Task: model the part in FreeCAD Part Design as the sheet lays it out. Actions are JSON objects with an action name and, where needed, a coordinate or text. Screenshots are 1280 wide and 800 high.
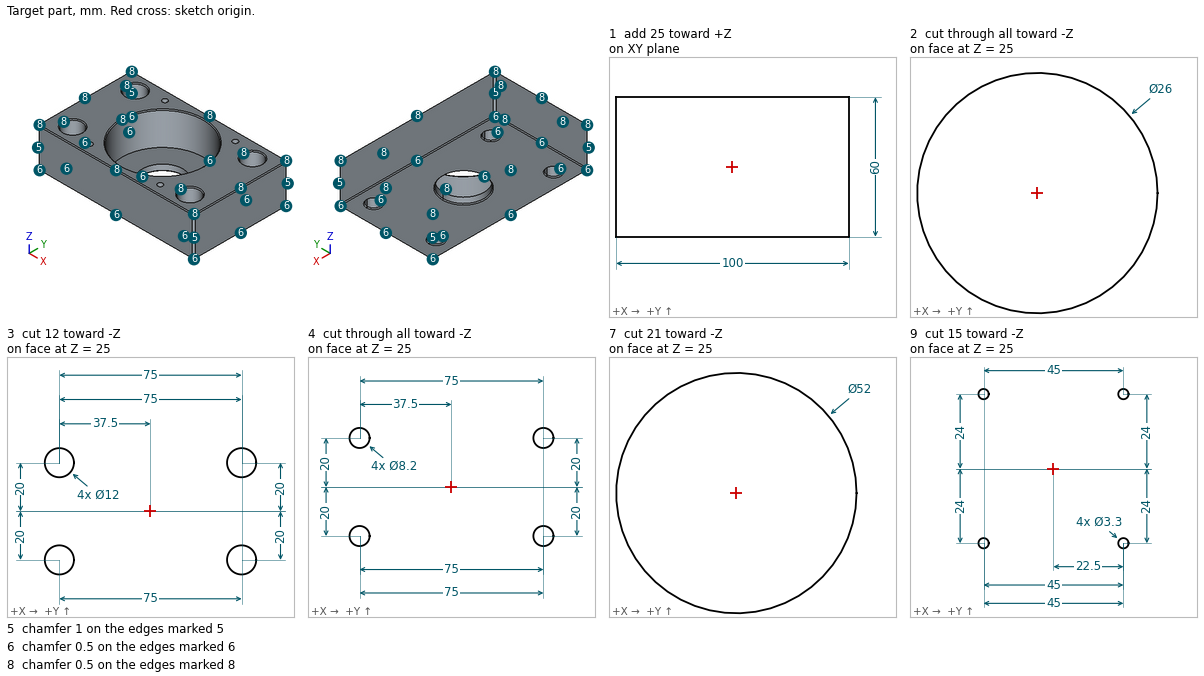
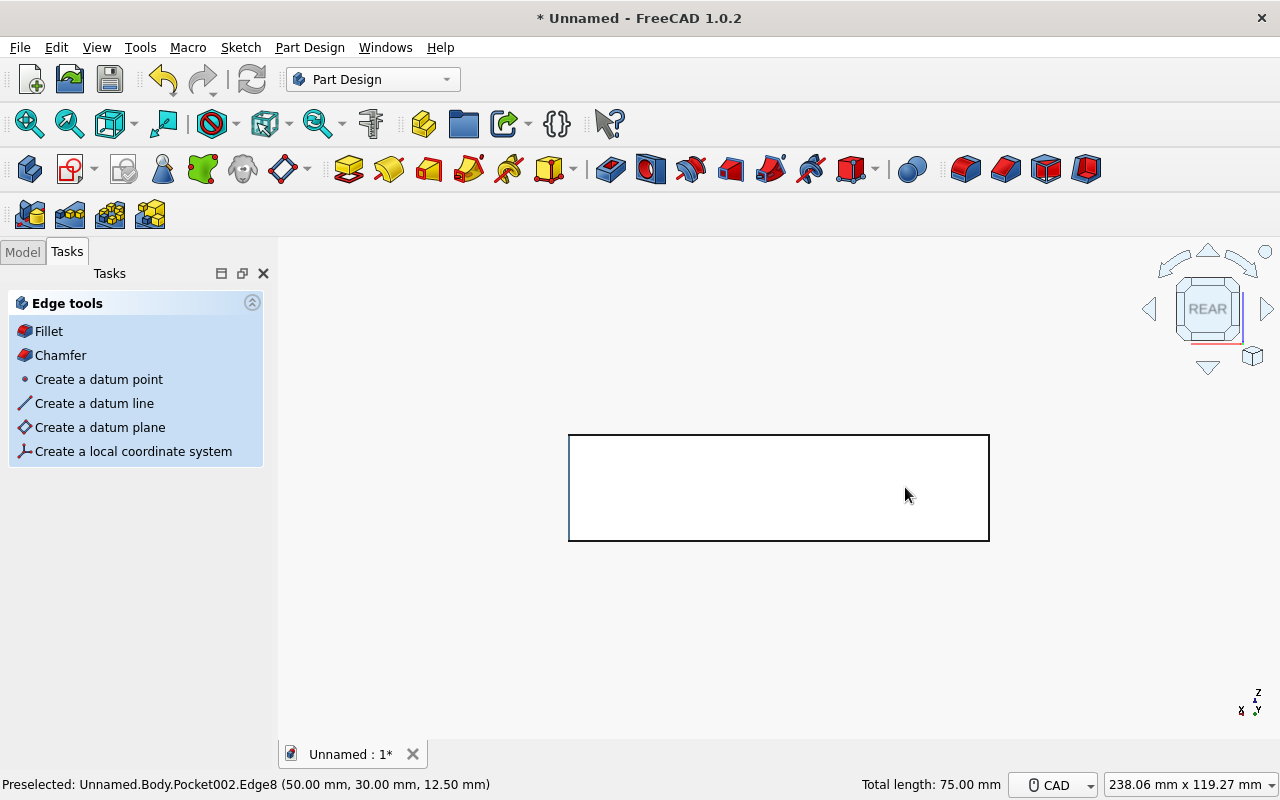
{"action": "key", "text": "v f"}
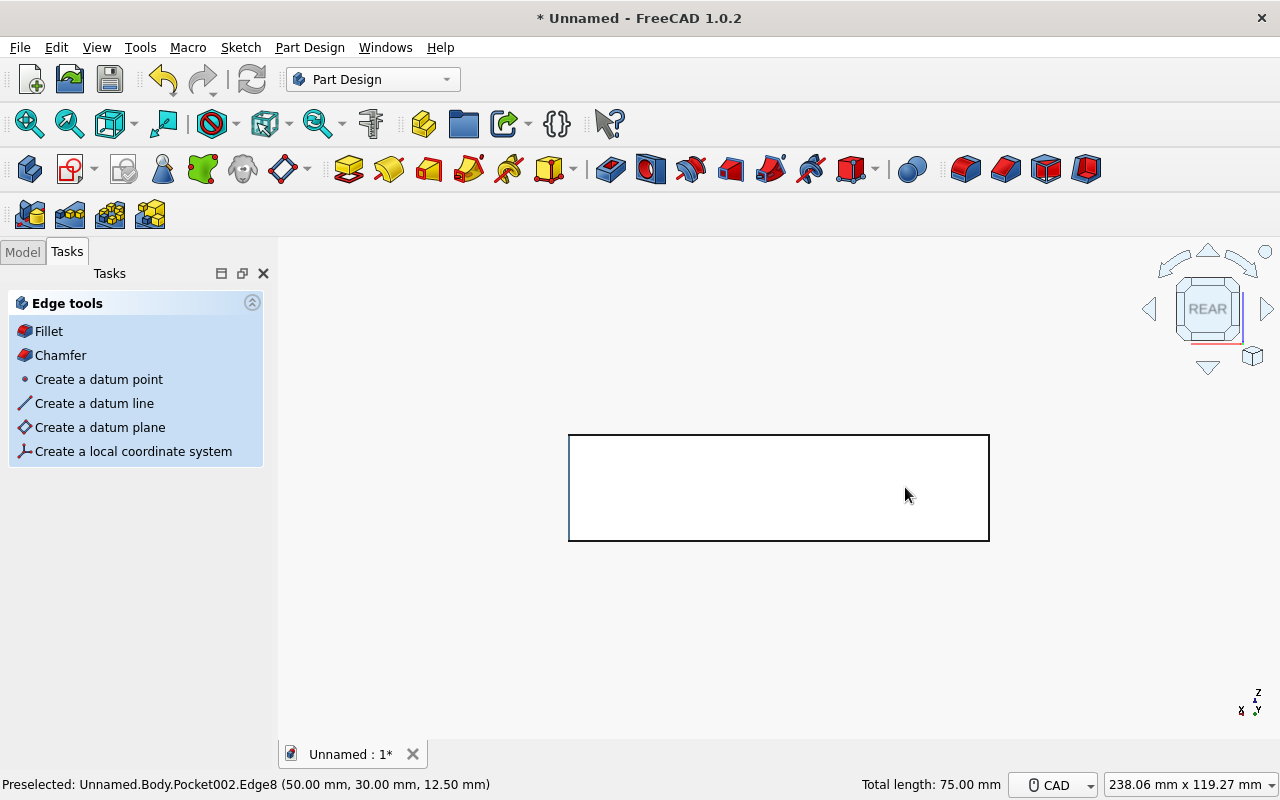
{"action": "left_click", "coordinate": [989, 487], "text": "ctrl"}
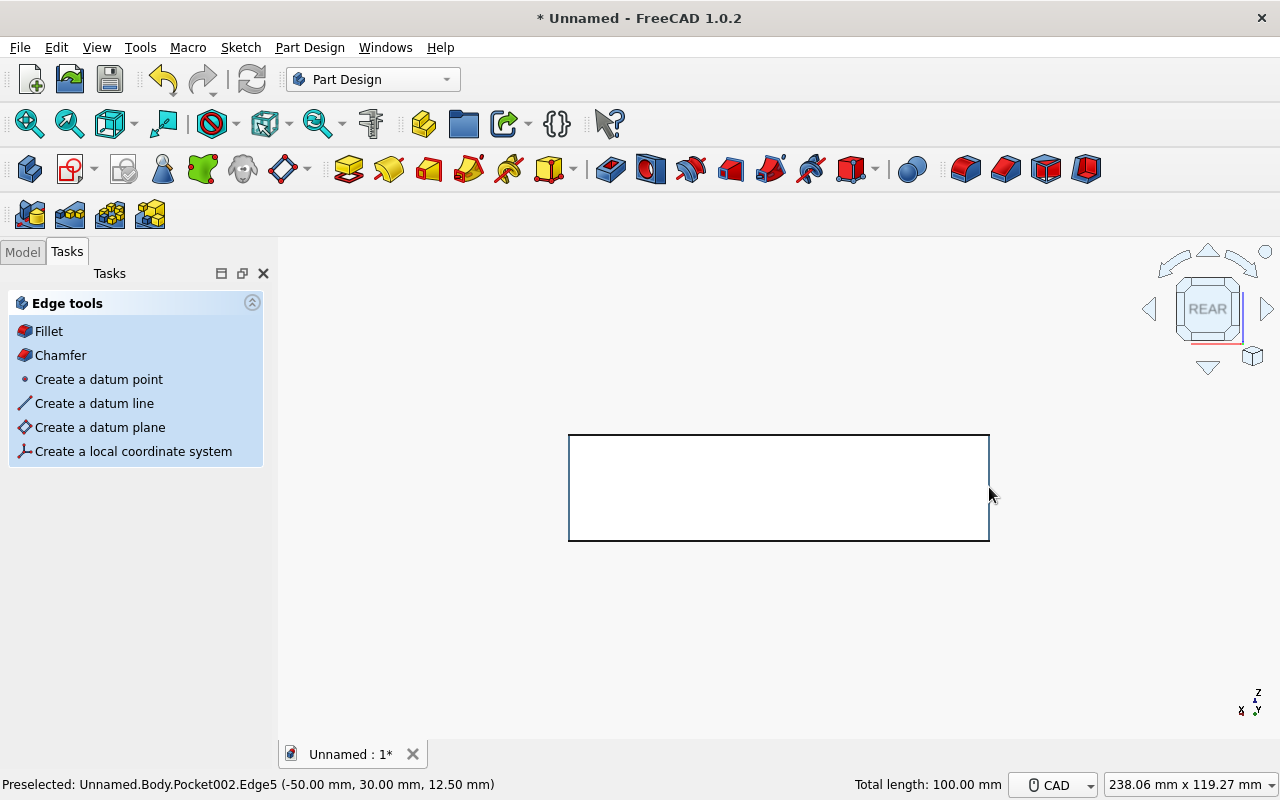
{"action": "left_click", "coordinate": [1006, 170]}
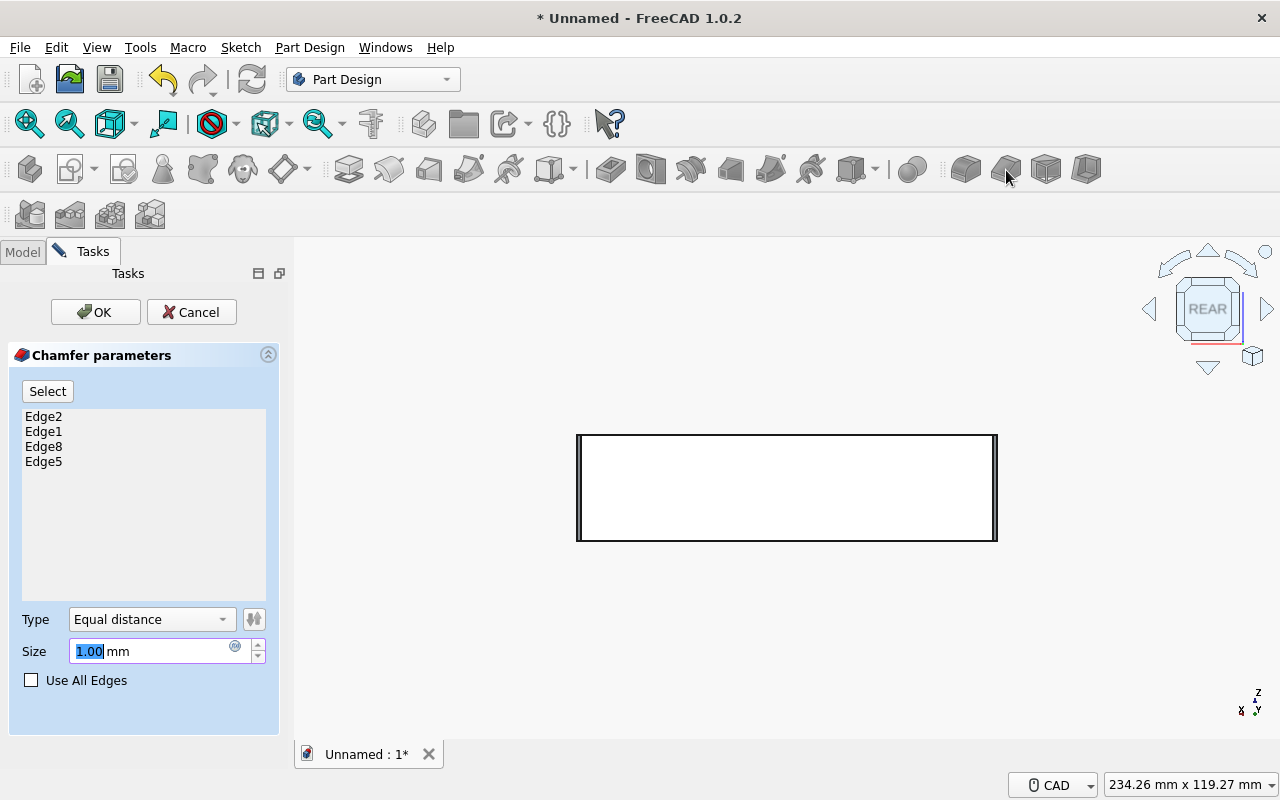
{"action": "type", "text": "1"}
{"action": "key", "text": "Tab"}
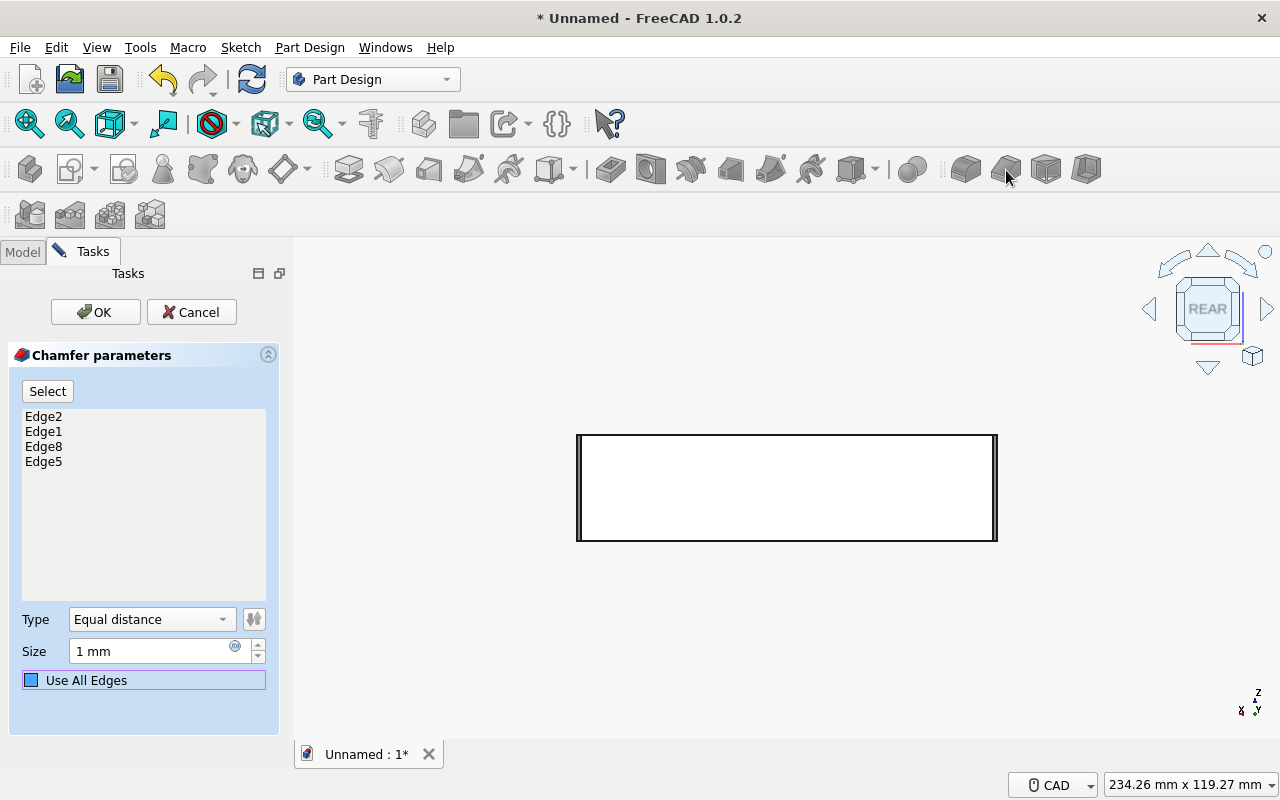
{"action": "left_click", "coordinate": [96, 312]}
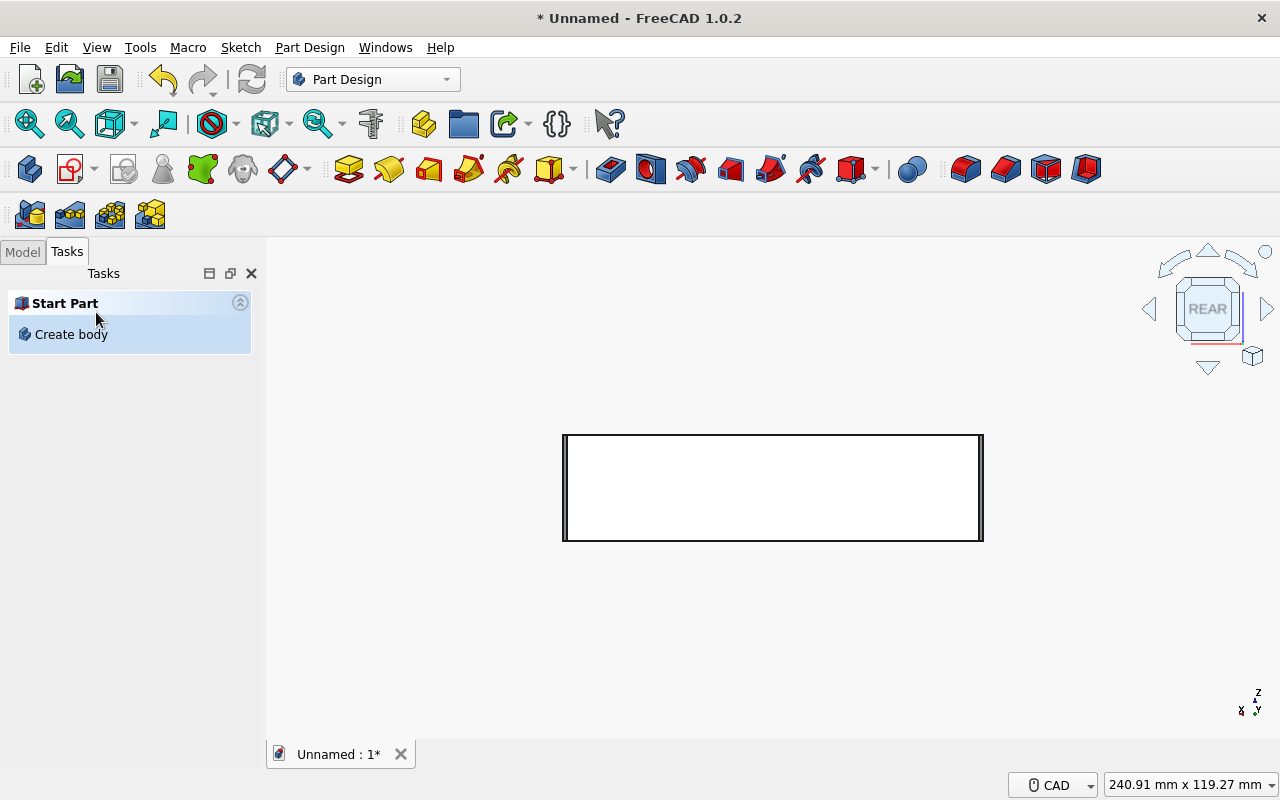
{"action": "left_click", "coordinate": [30, 124]}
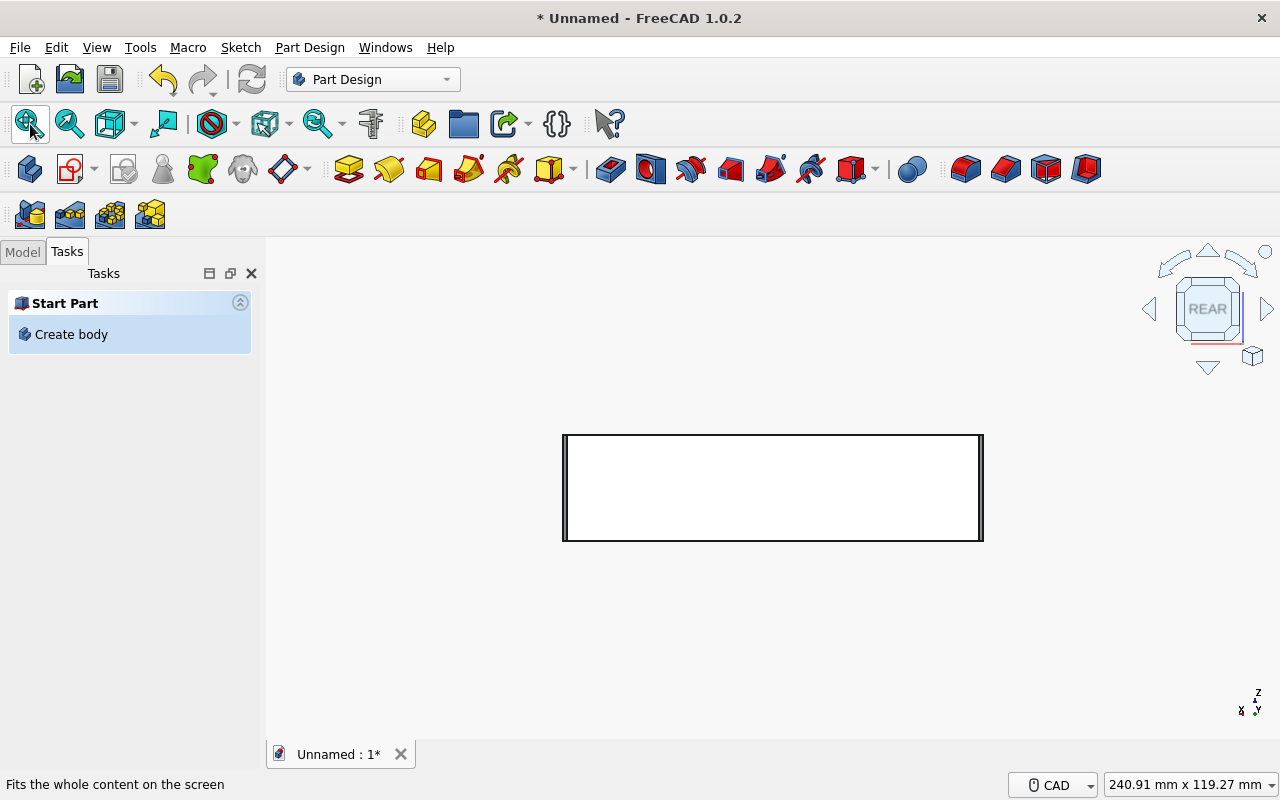
{"action": "key", "text": "0"}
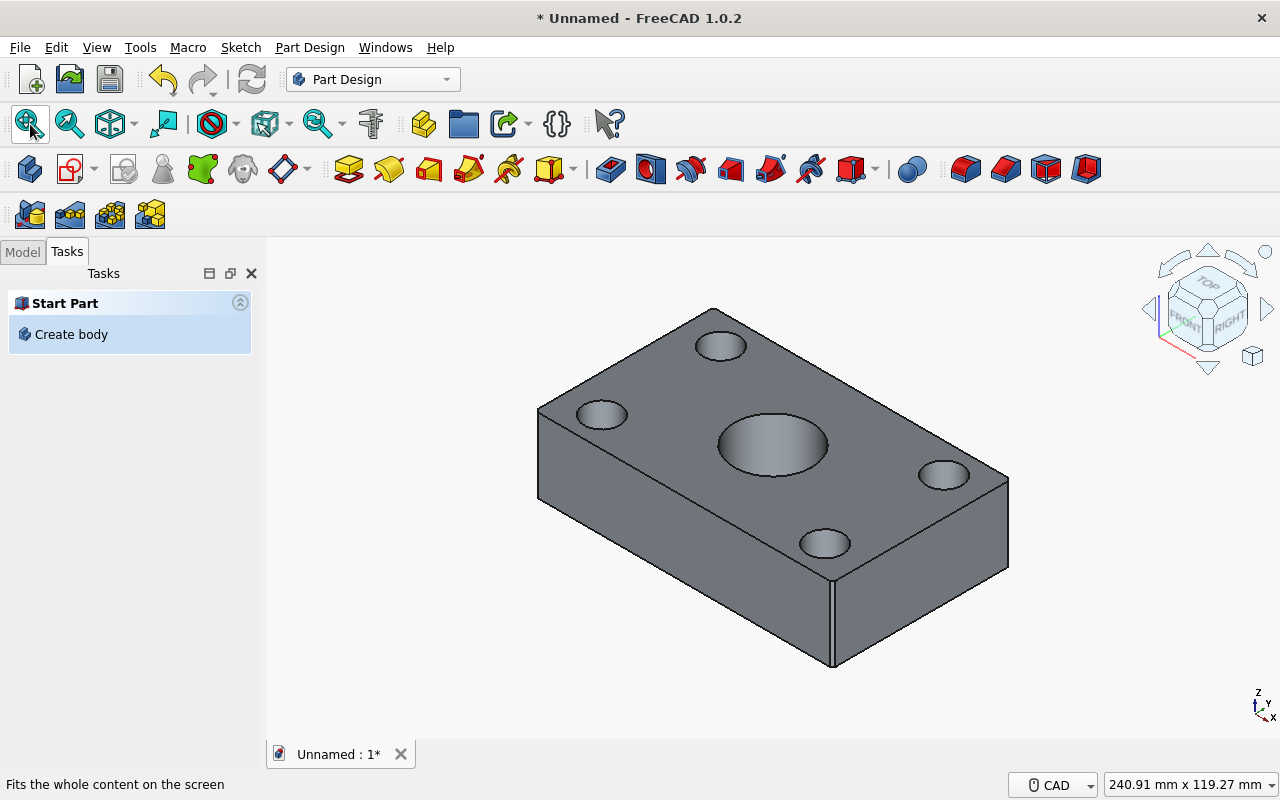
{"action": "key", "text": "2"}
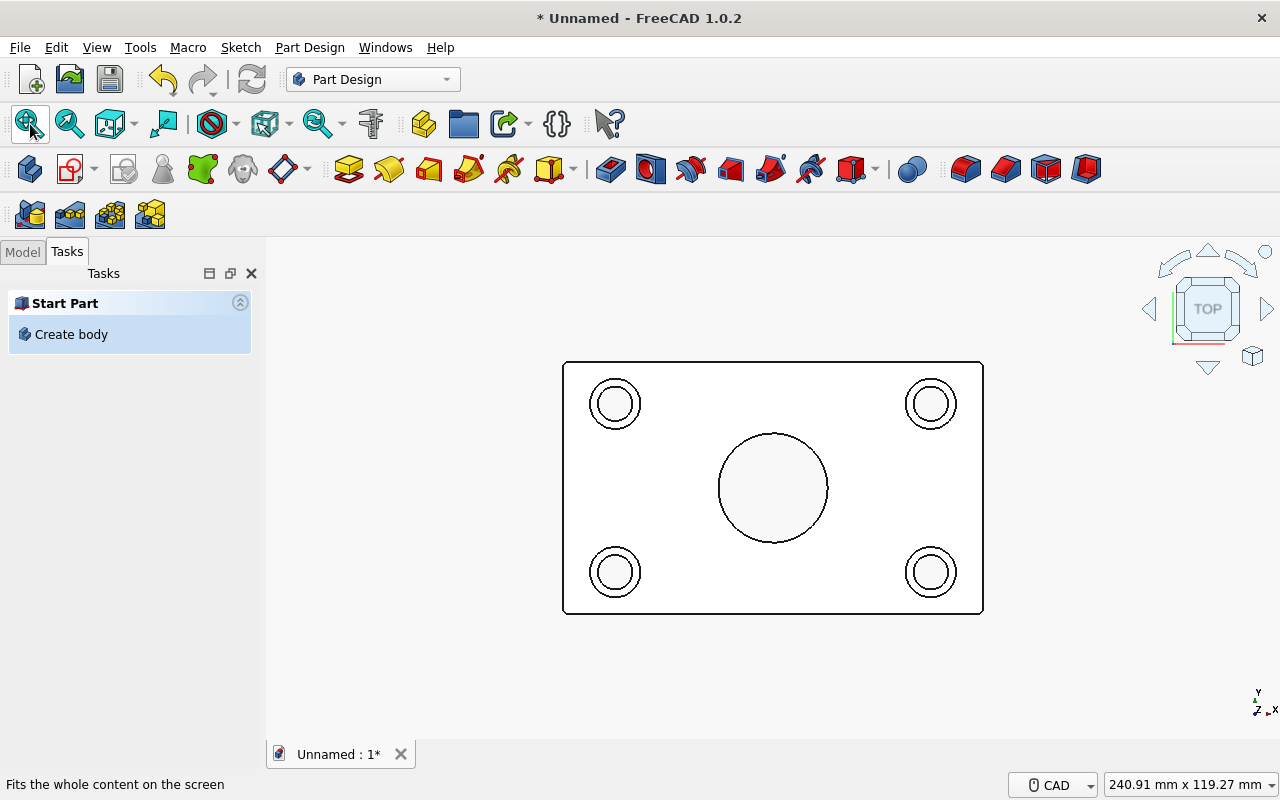
{"action": "key", "text": "1"}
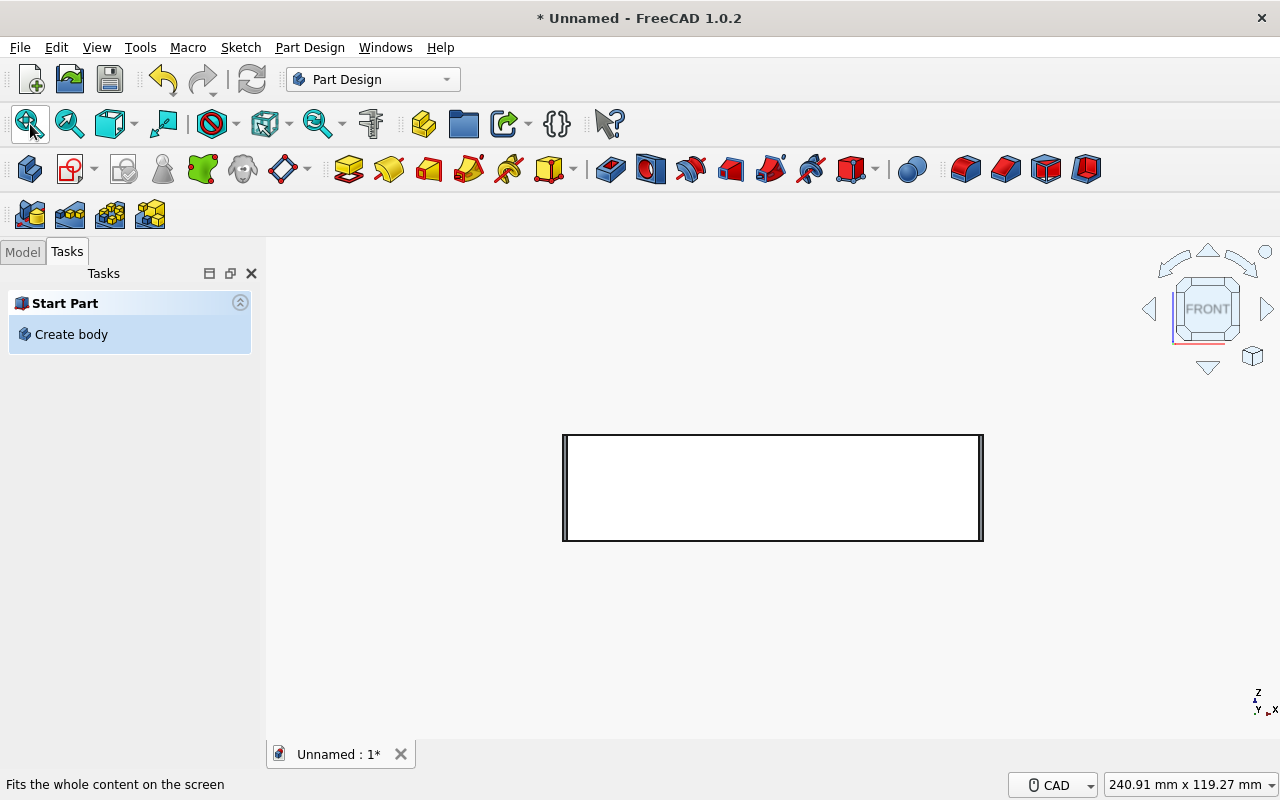
{"action": "key", "text": "v f"}